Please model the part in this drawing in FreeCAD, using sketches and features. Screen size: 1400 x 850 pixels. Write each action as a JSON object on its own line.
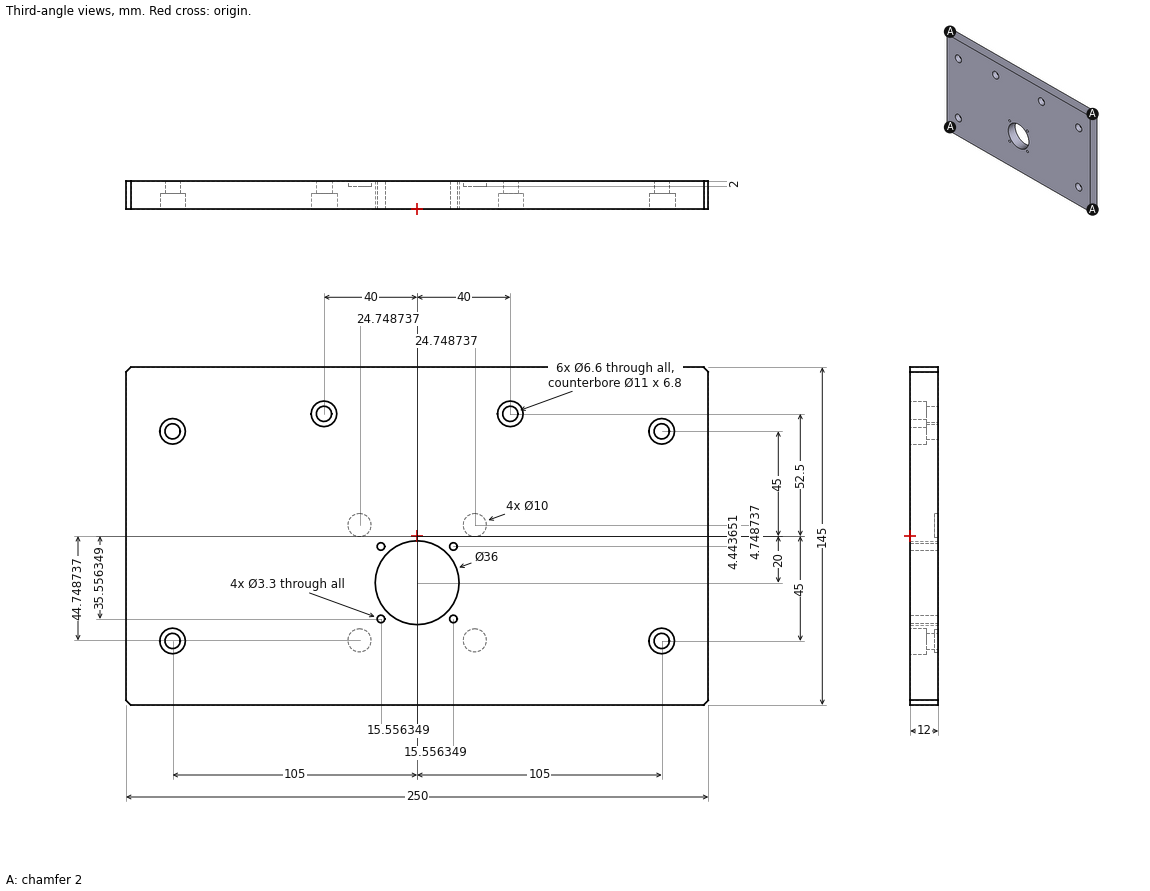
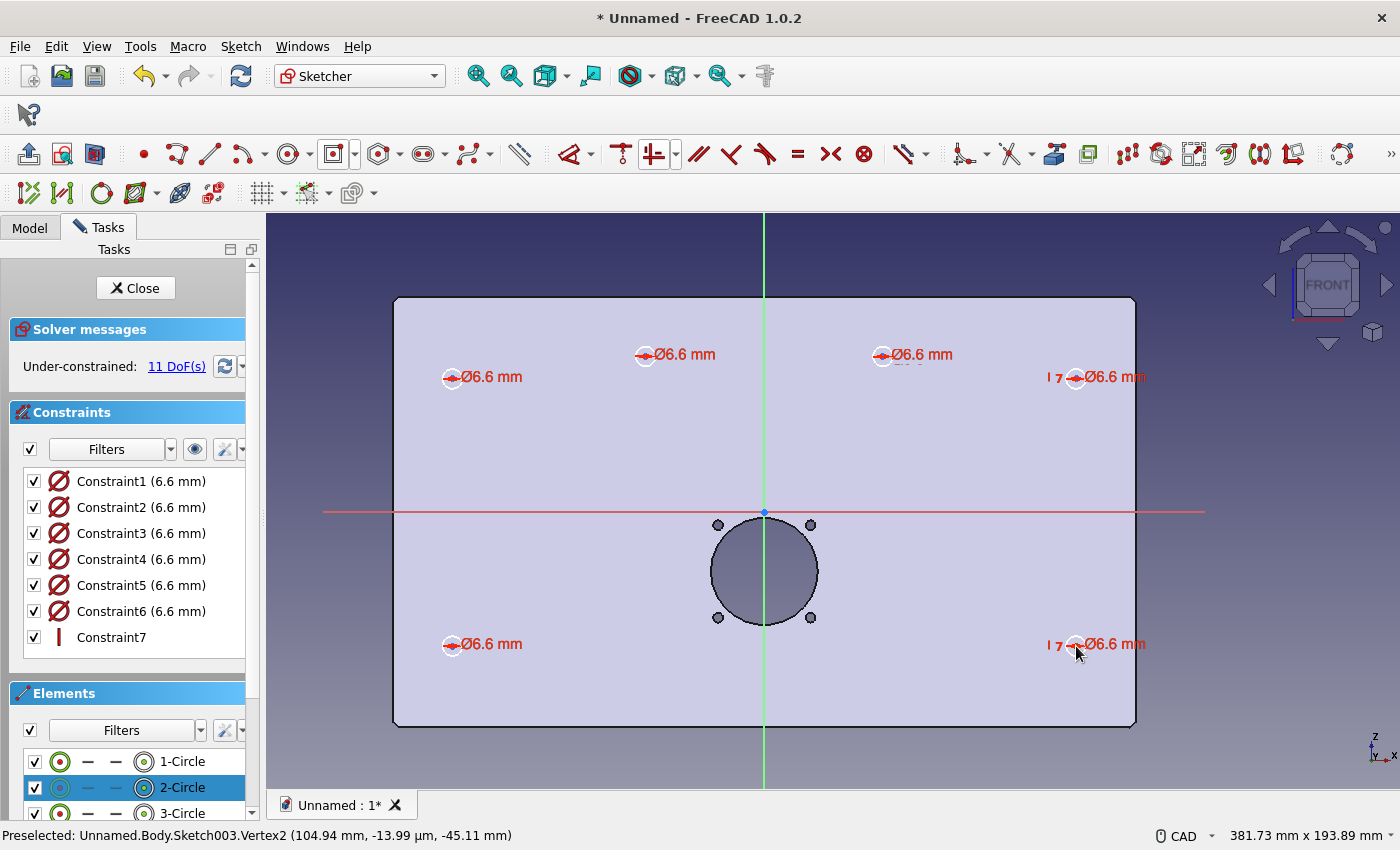
{"action": "left_click", "coordinate": [452, 646]}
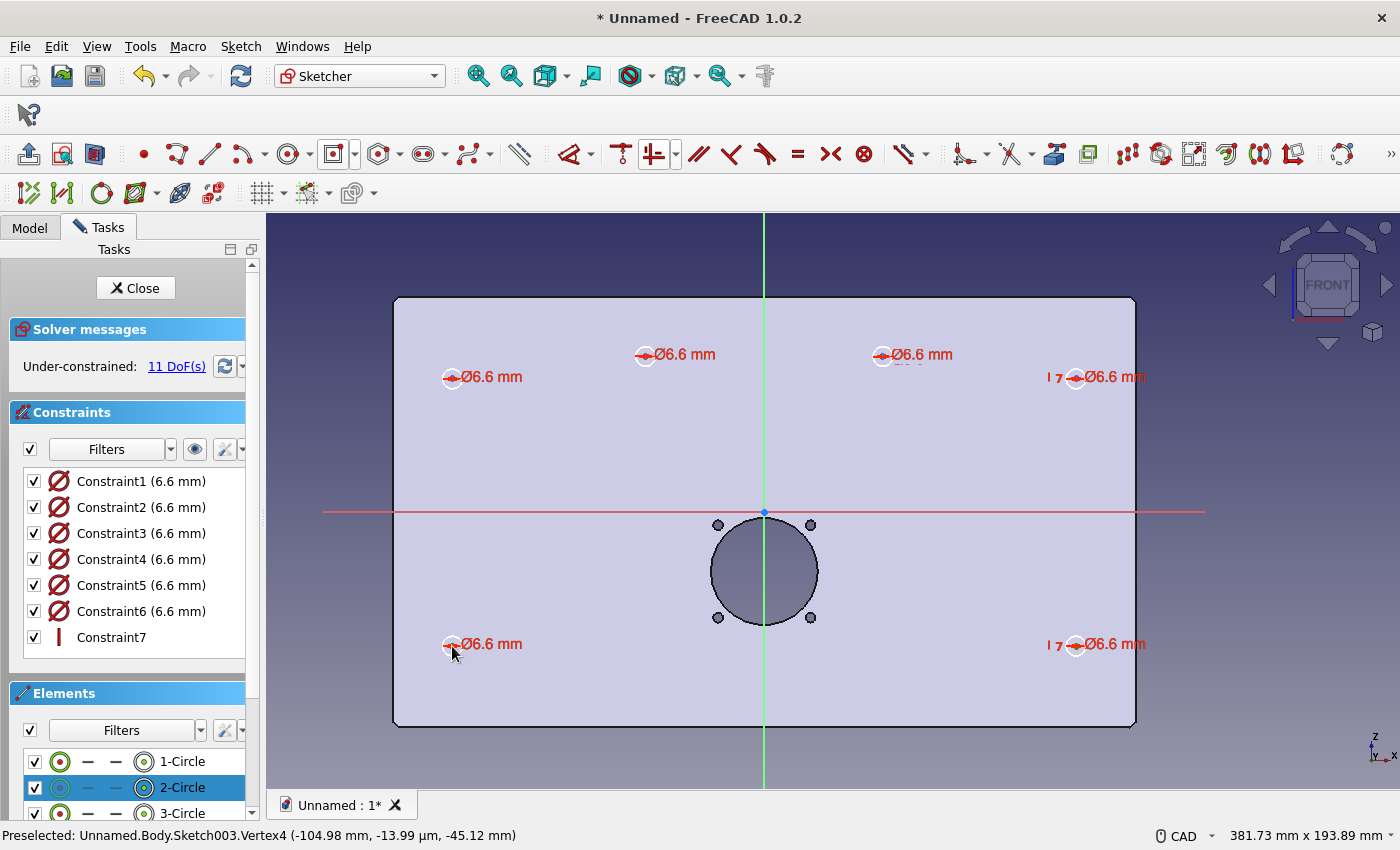
{"action": "key", "text": "h"}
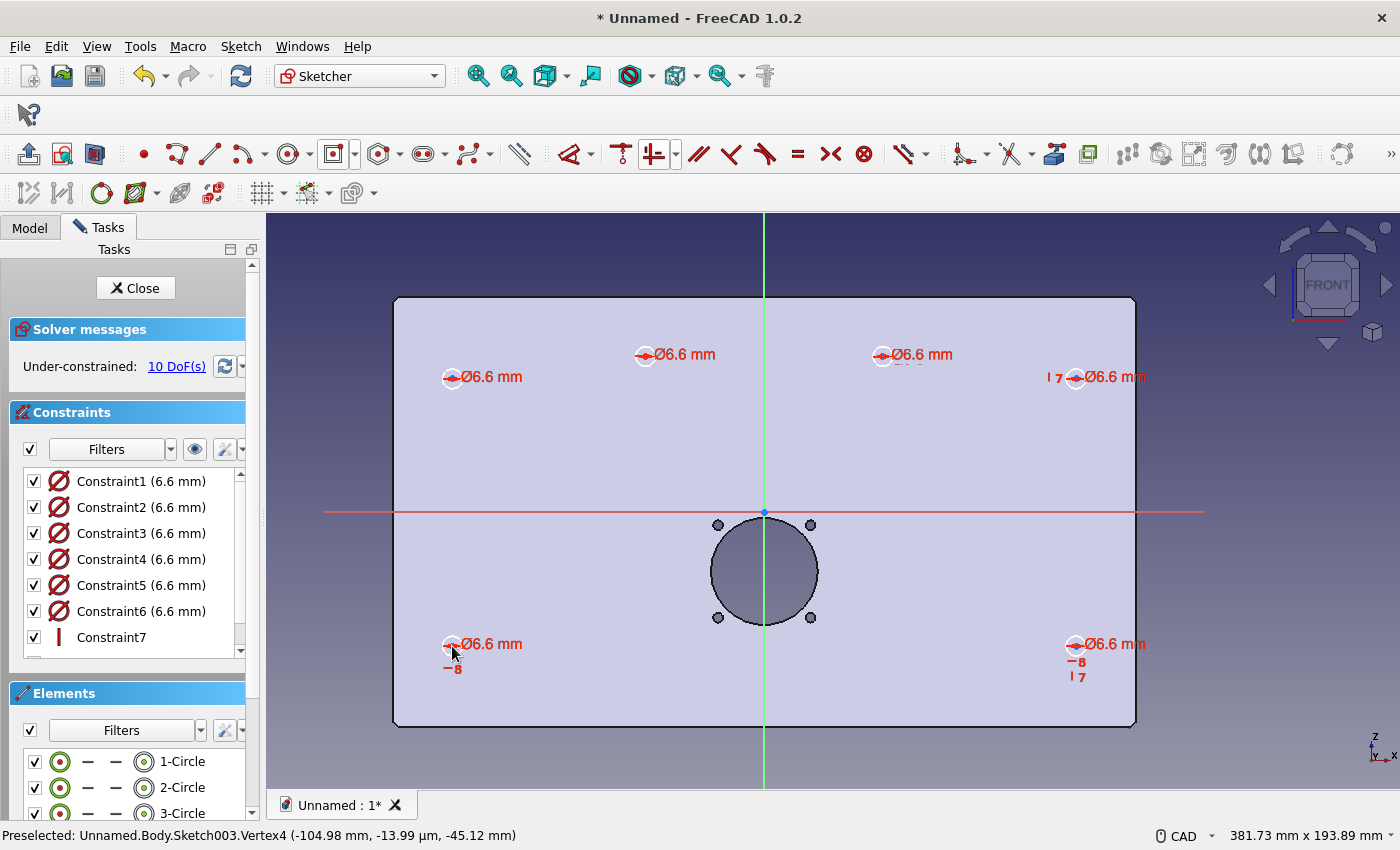
{"action": "left_click", "coordinate": [452, 646]}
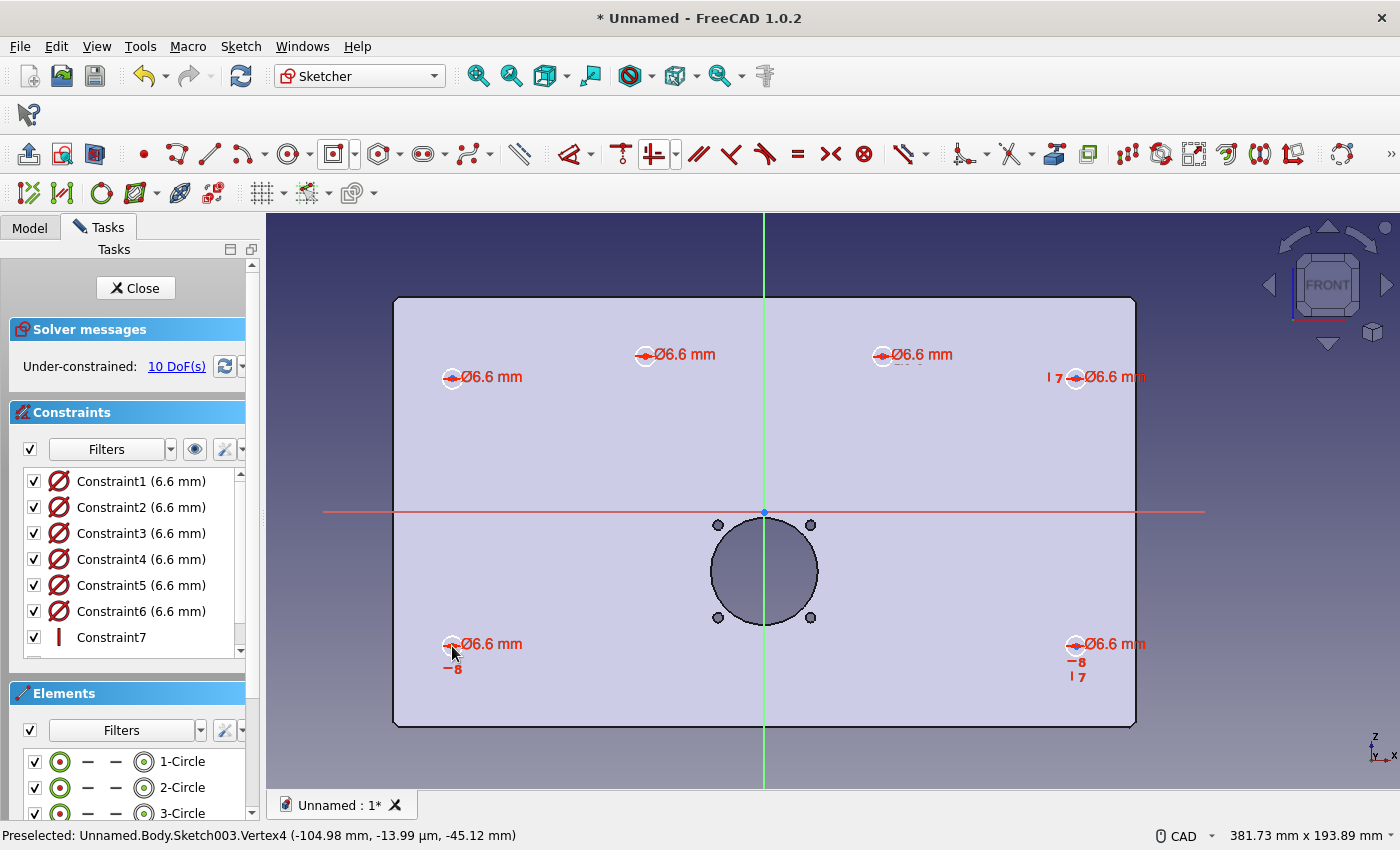
{"action": "left_click", "coordinate": [452, 379]}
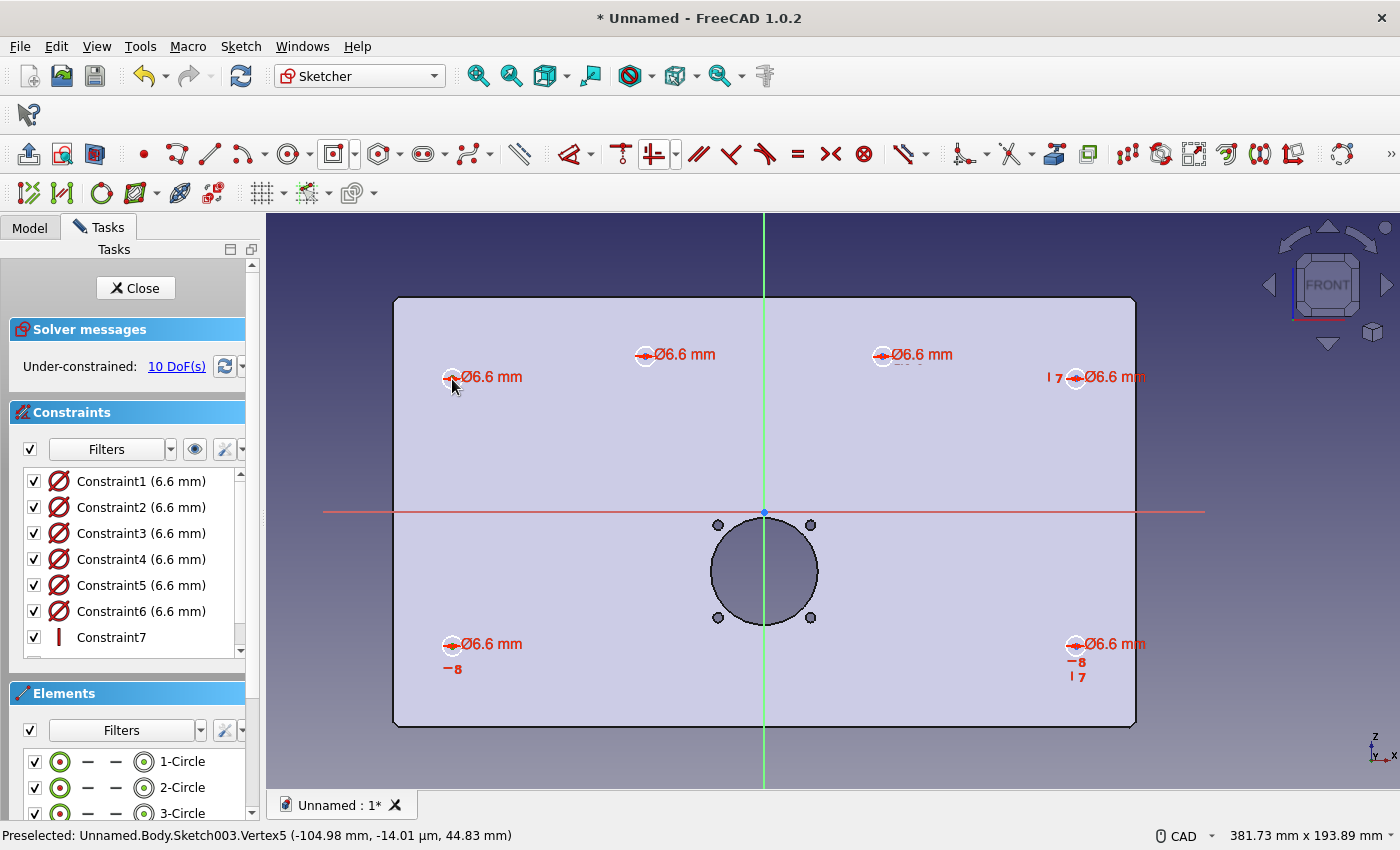
{"action": "left_click", "coordinate": [676, 154]}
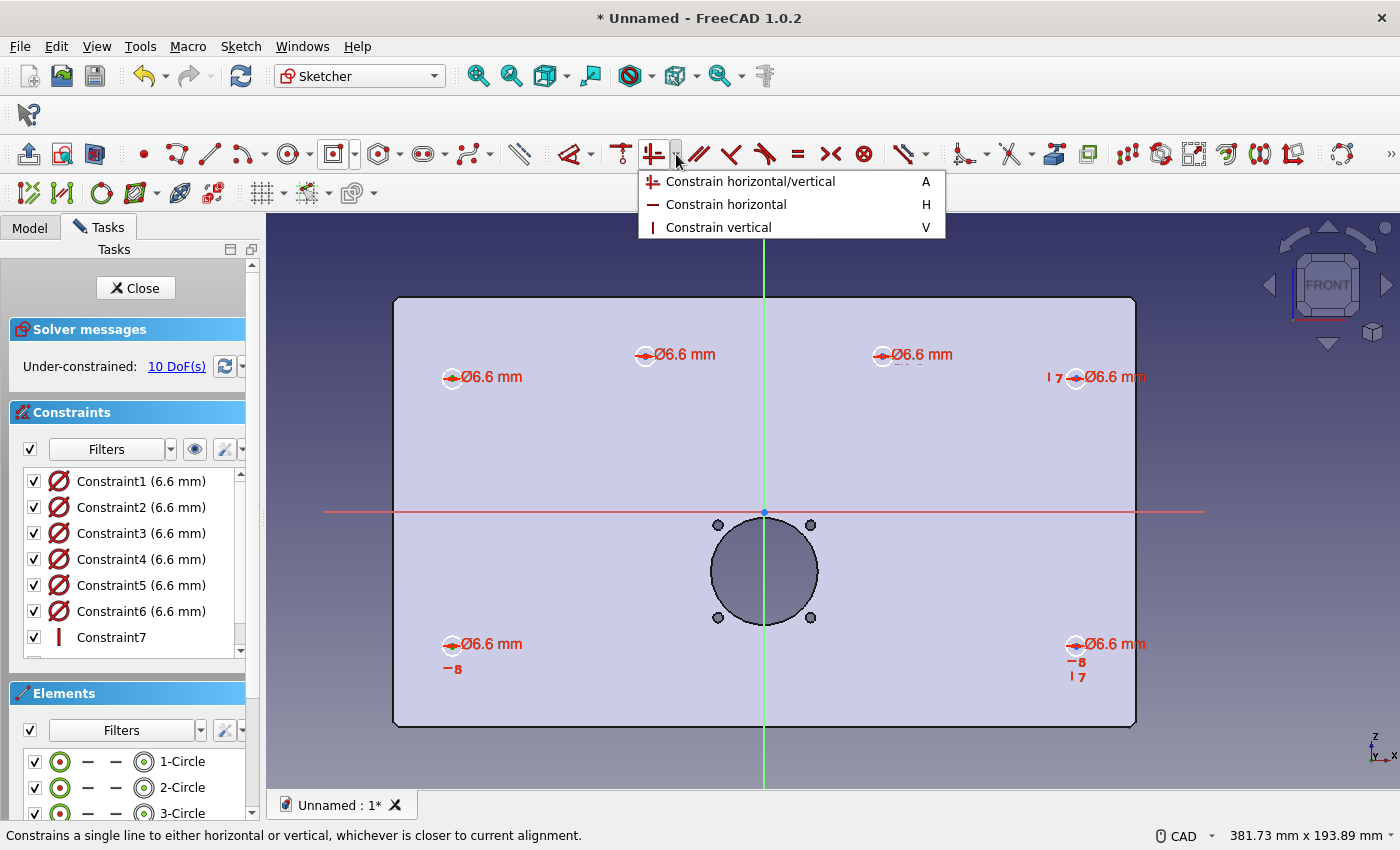
{"action": "left_click", "coordinate": [792, 228]}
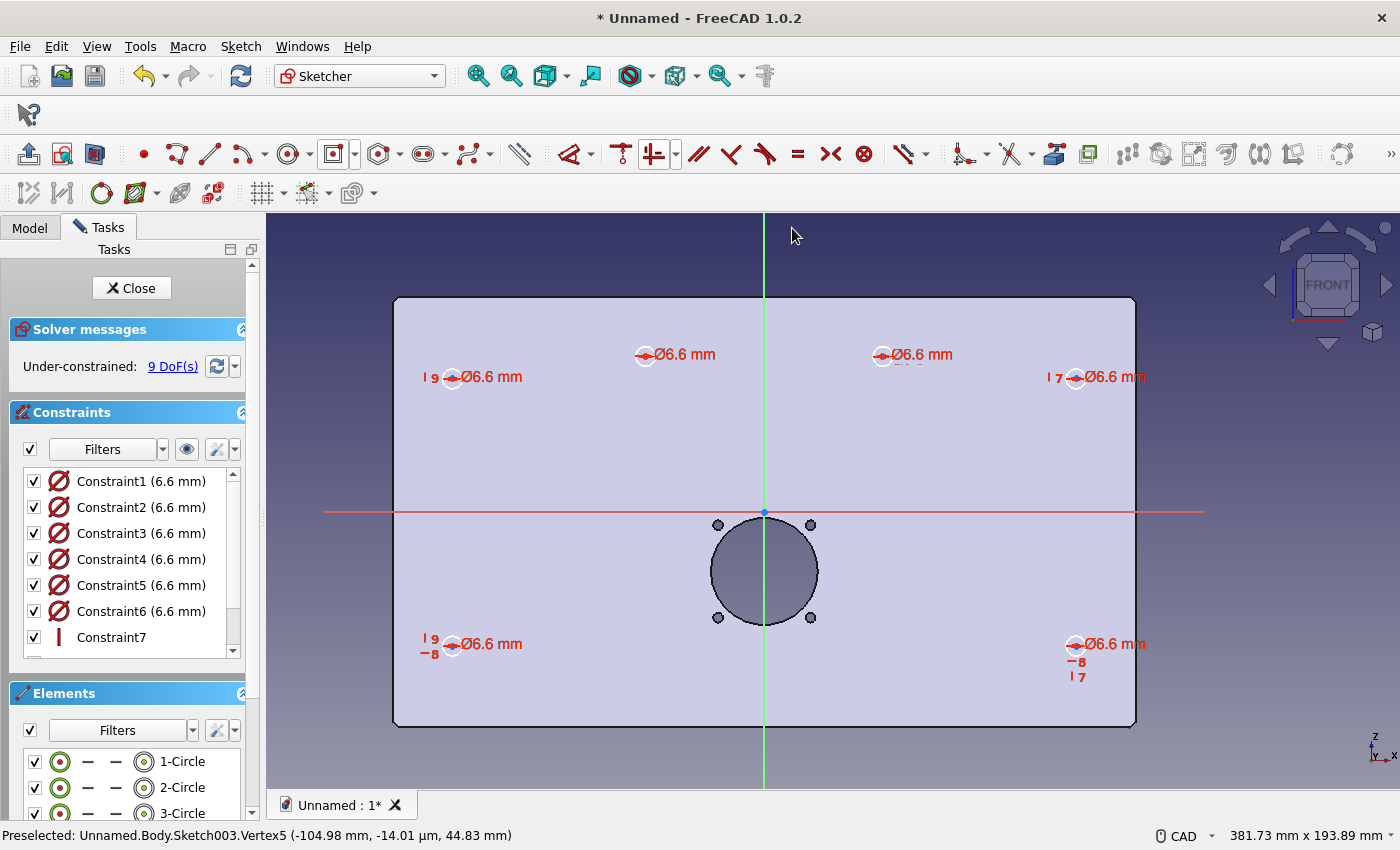
{"action": "left_click", "coordinate": [1076, 379]}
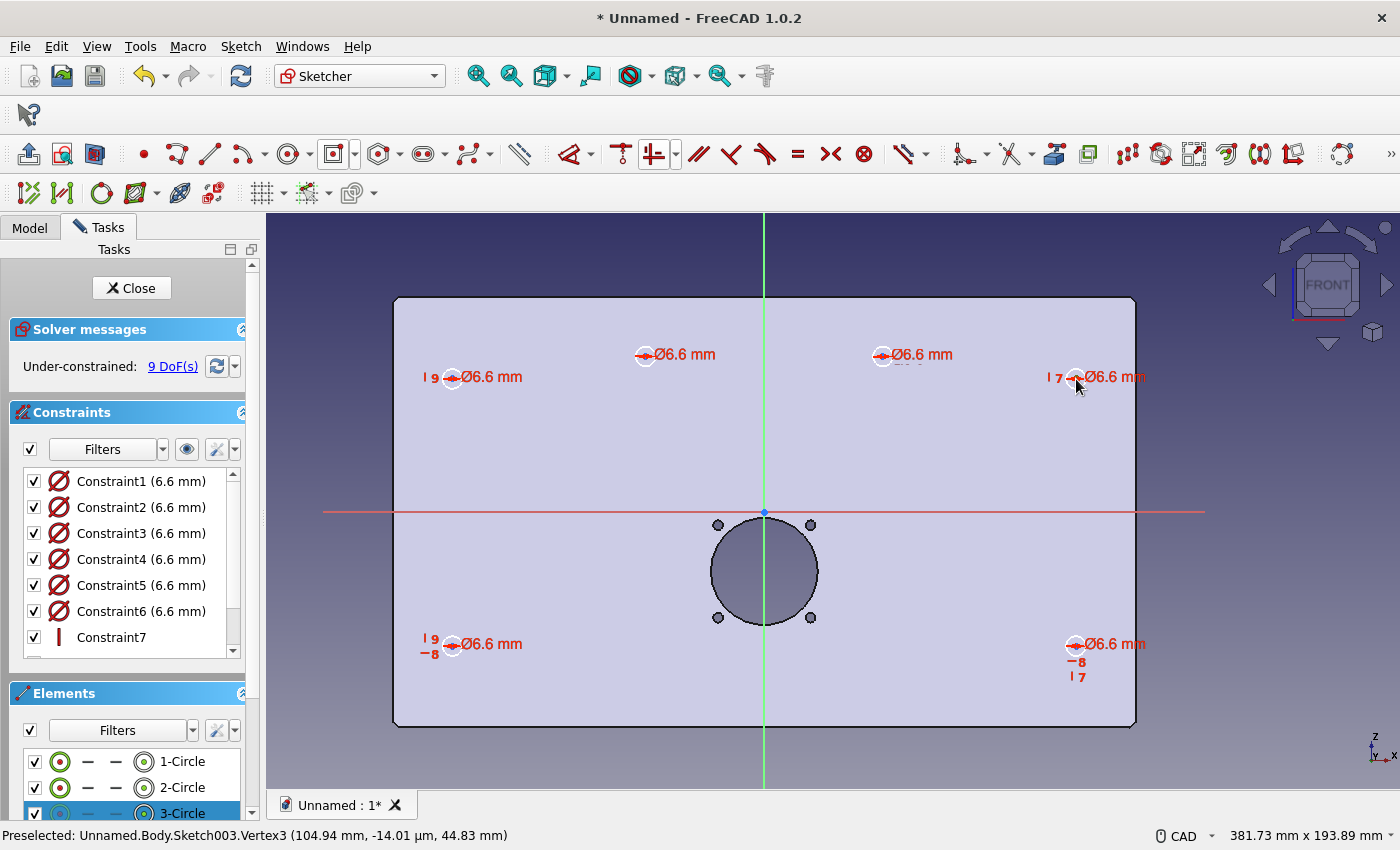
{"action": "left_click", "coordinate": [452, 379]}